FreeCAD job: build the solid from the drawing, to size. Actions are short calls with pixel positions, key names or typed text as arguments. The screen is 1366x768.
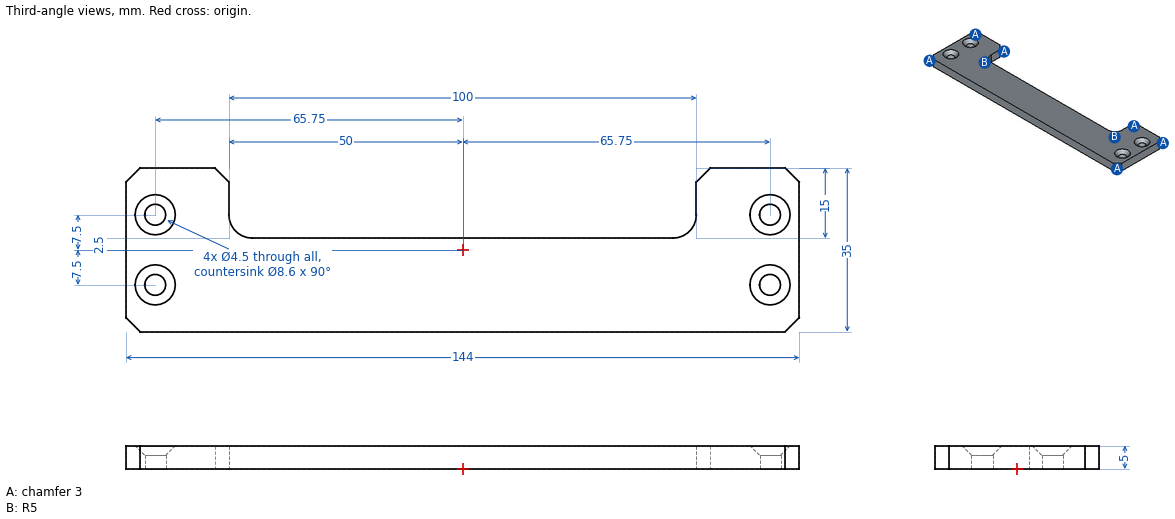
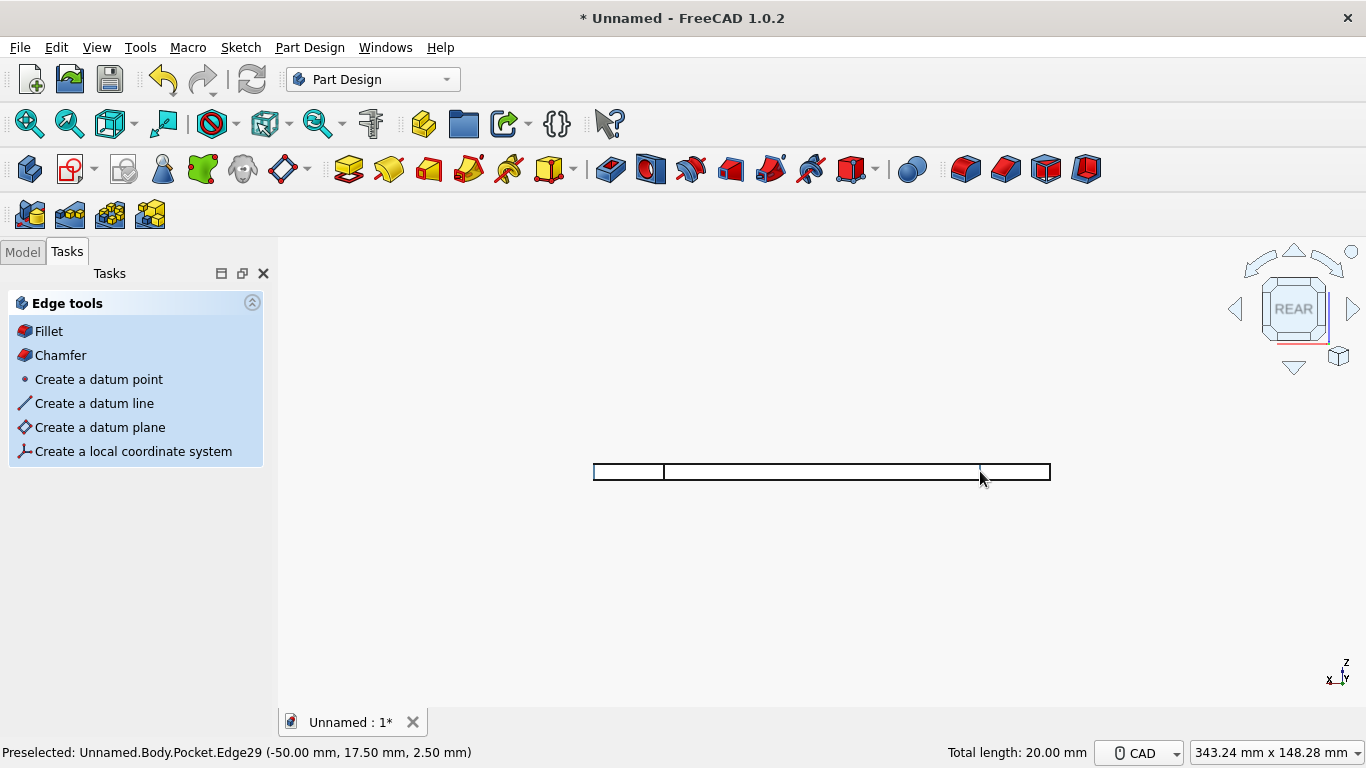
click(664, 471, ctrl)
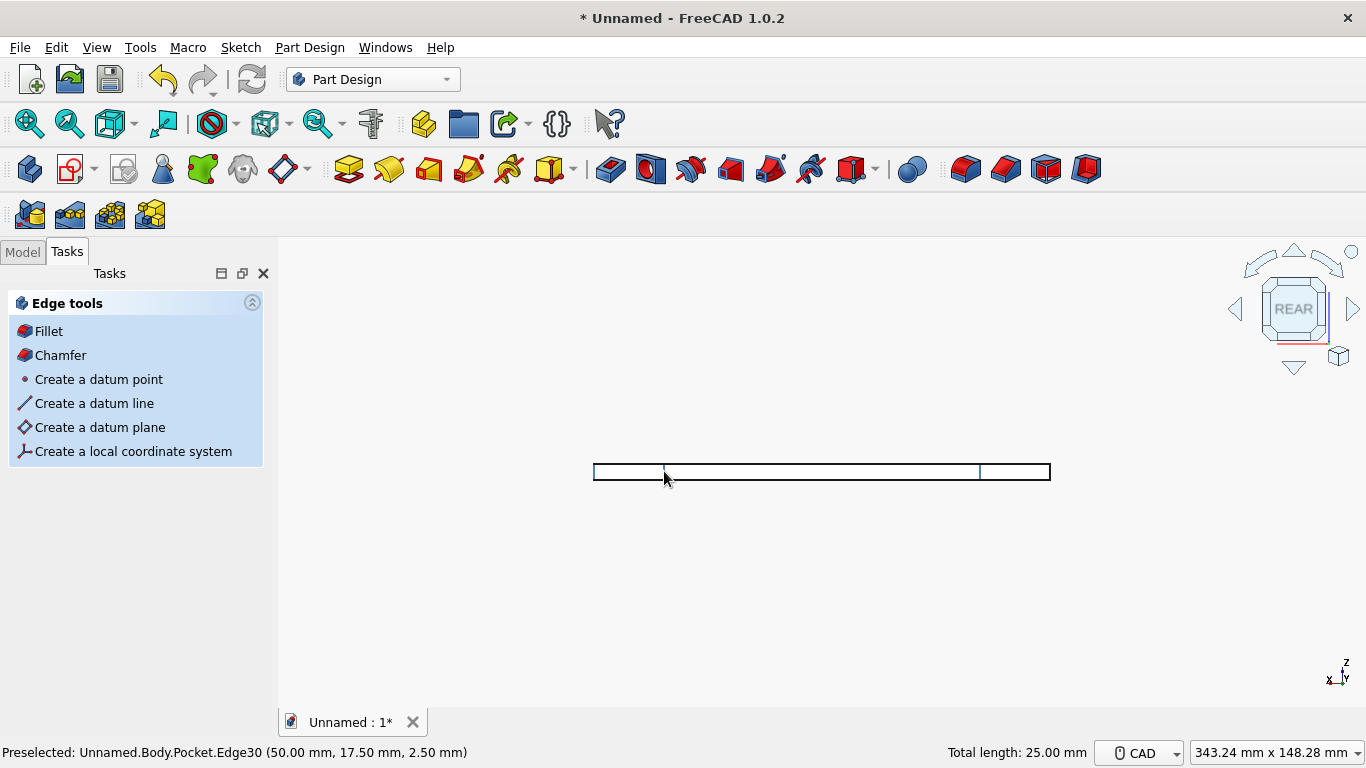
click(1050, 471, ctrl)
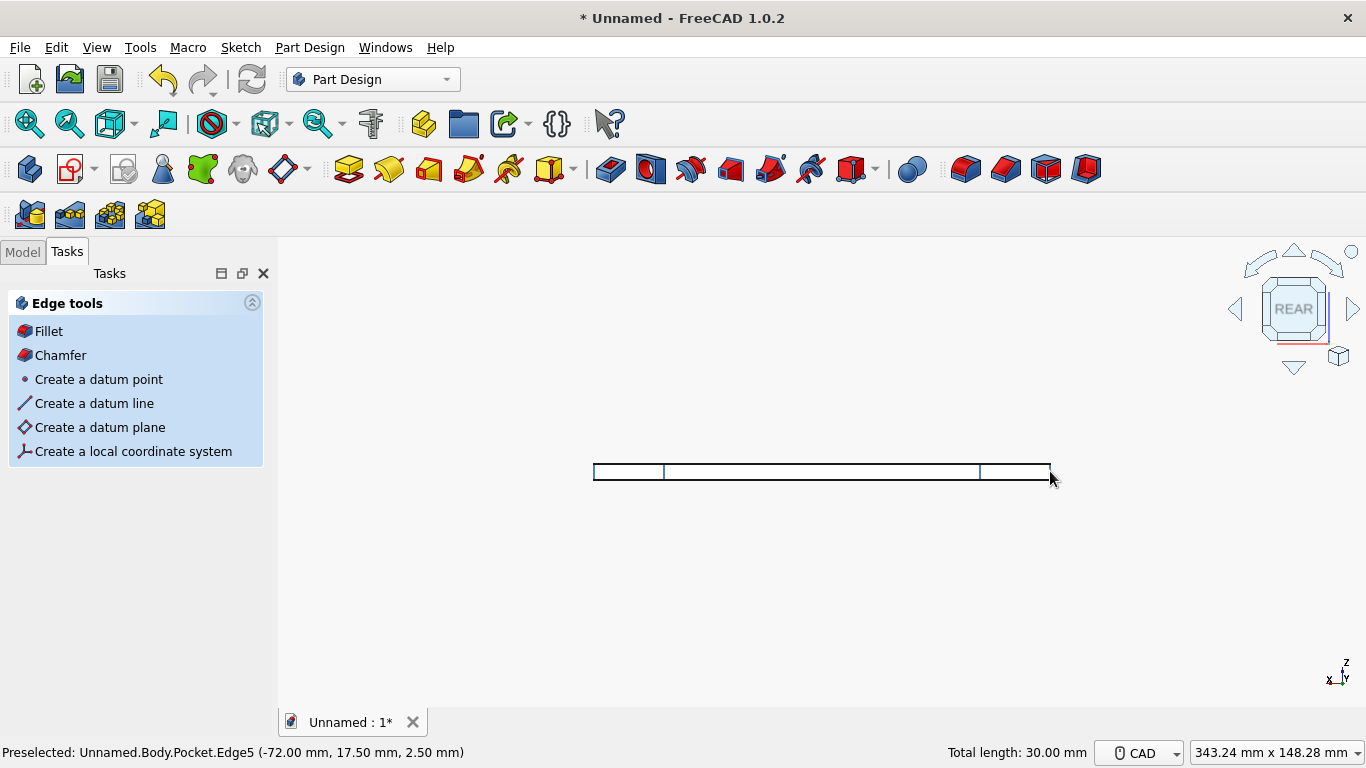
click(1006, 170)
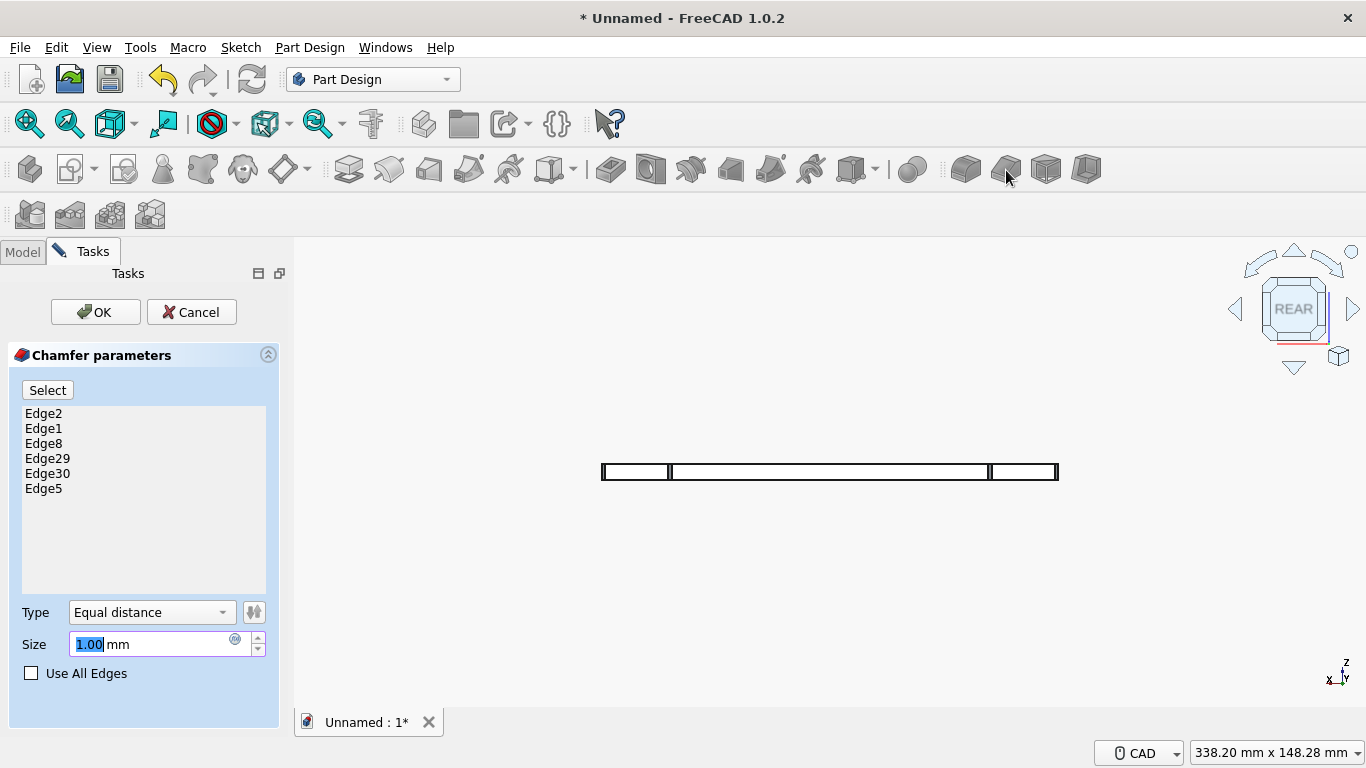
text(3)
key(Tab)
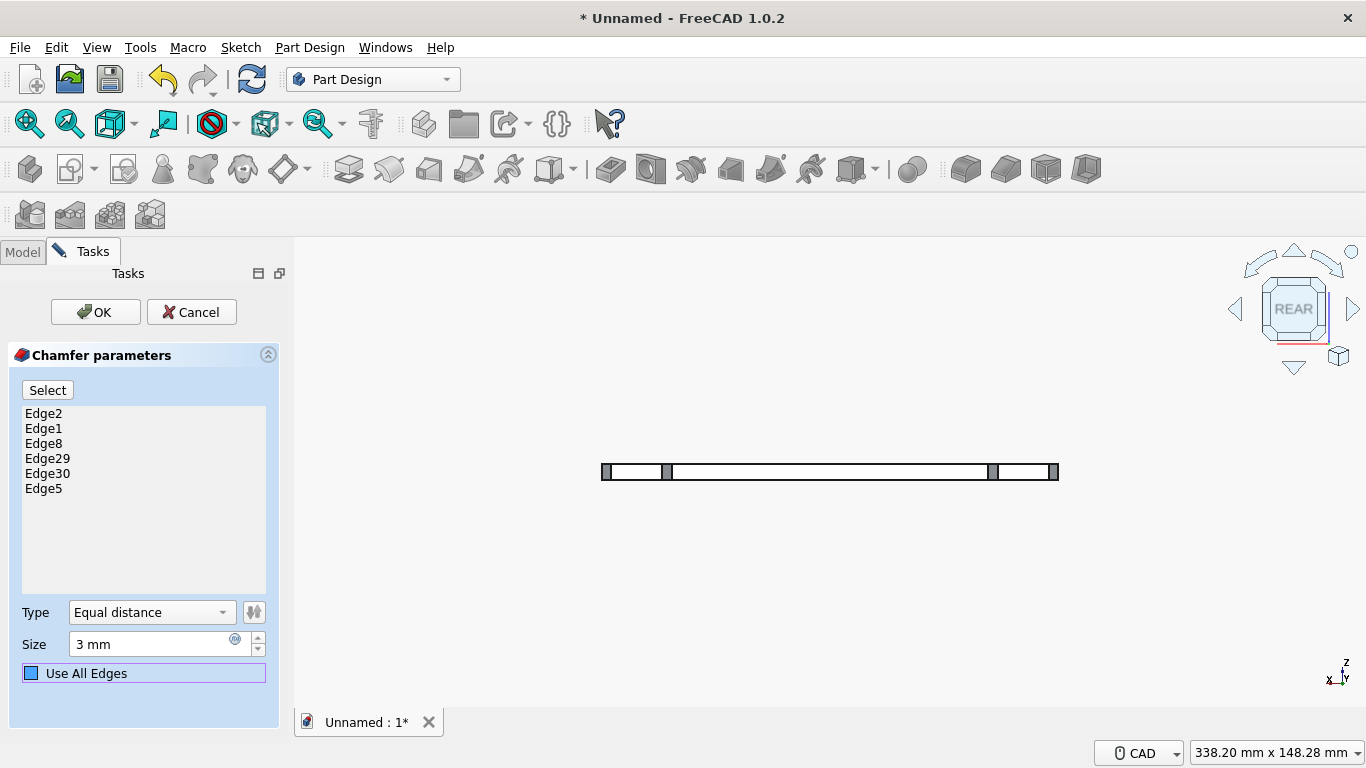
click(96, 312)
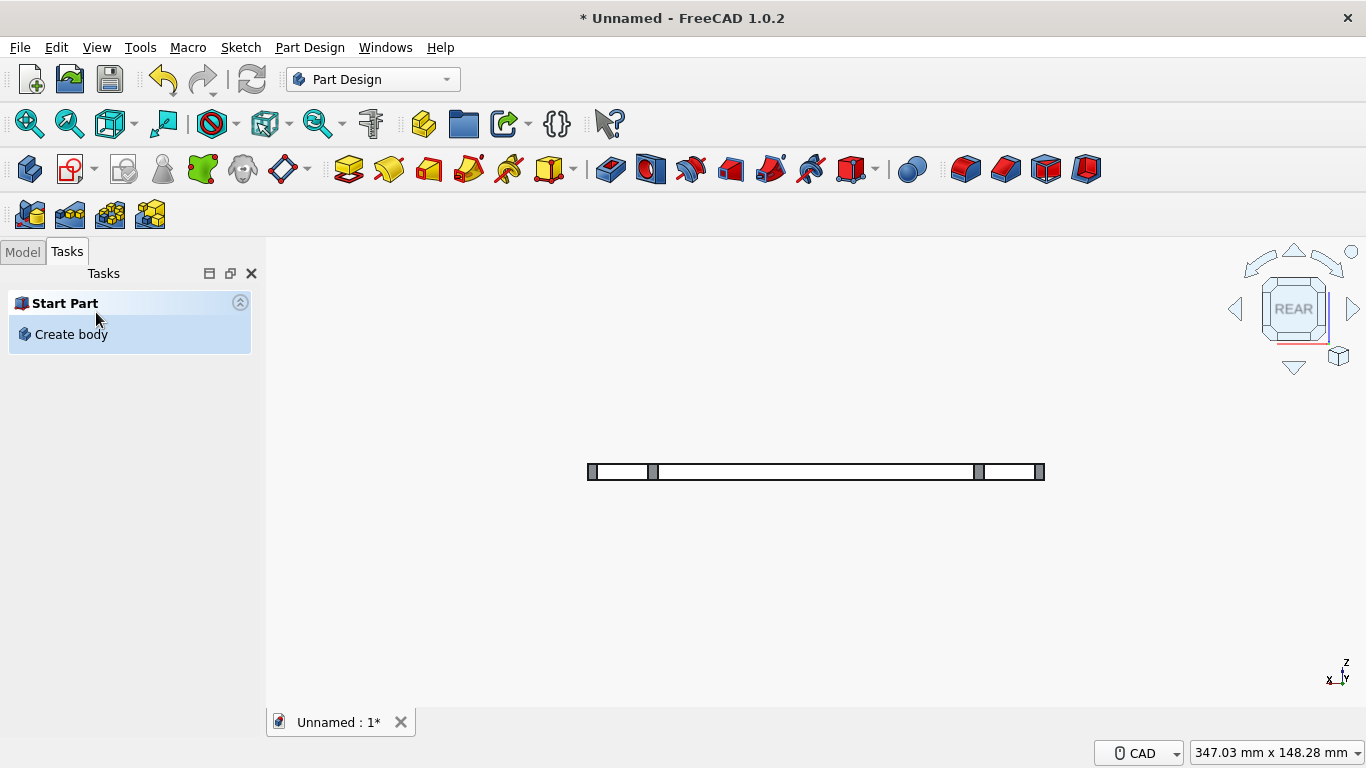
key(v)
key(f)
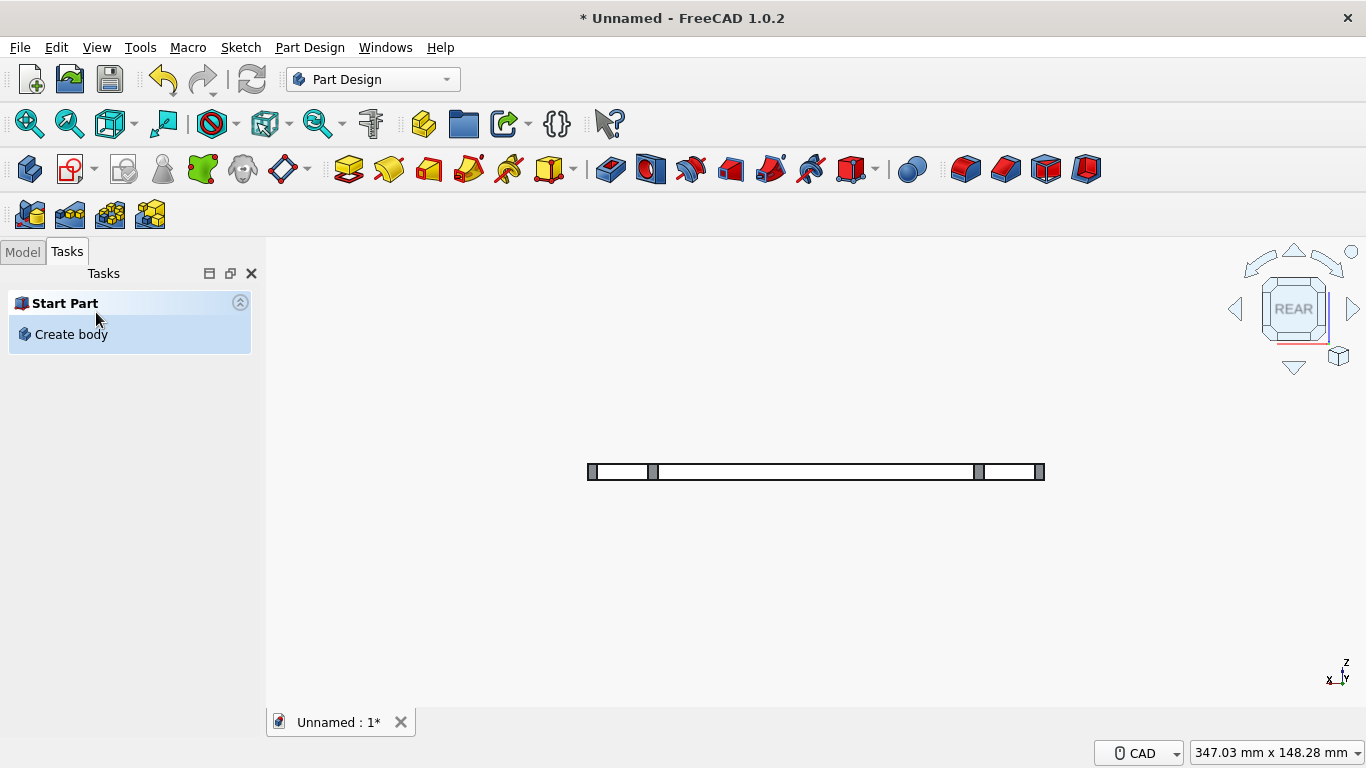
scroll(974, 471, up, 5)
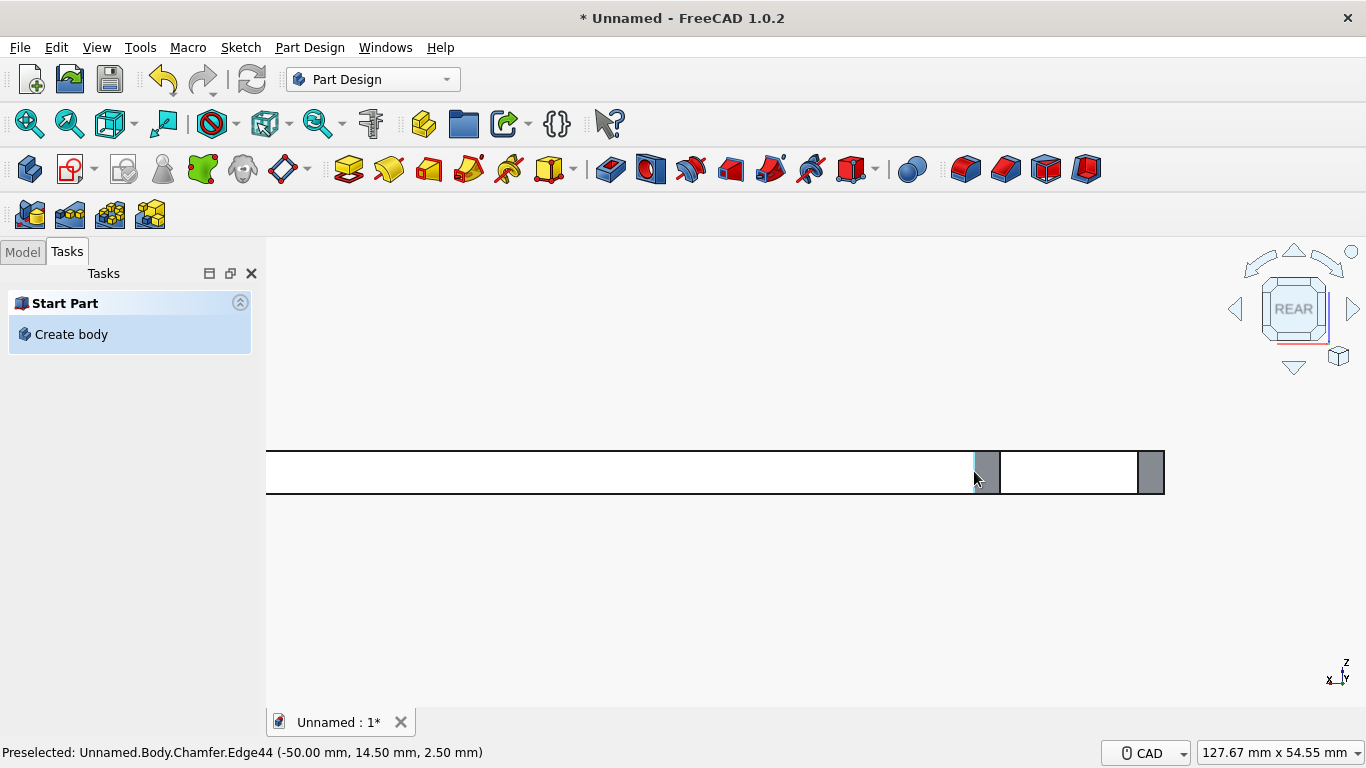
key(v)
key(f)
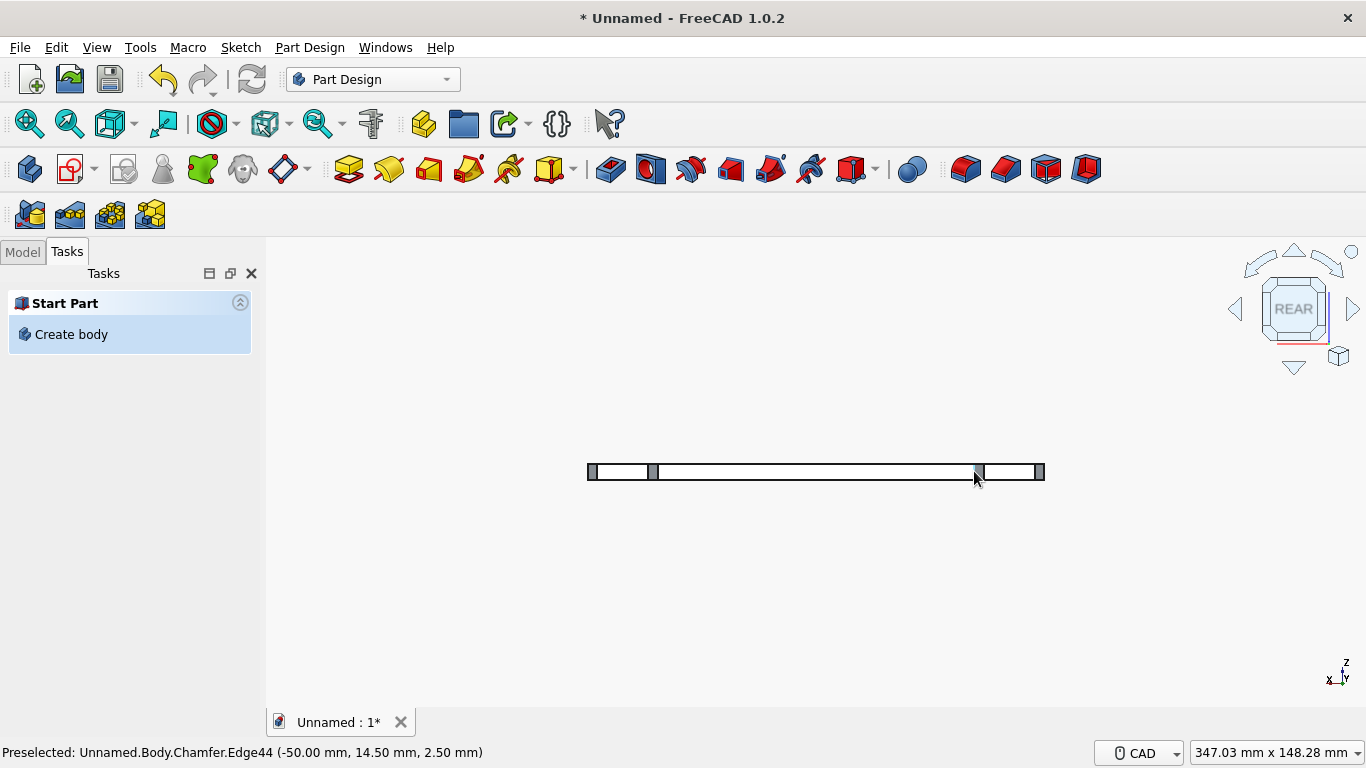
key(0)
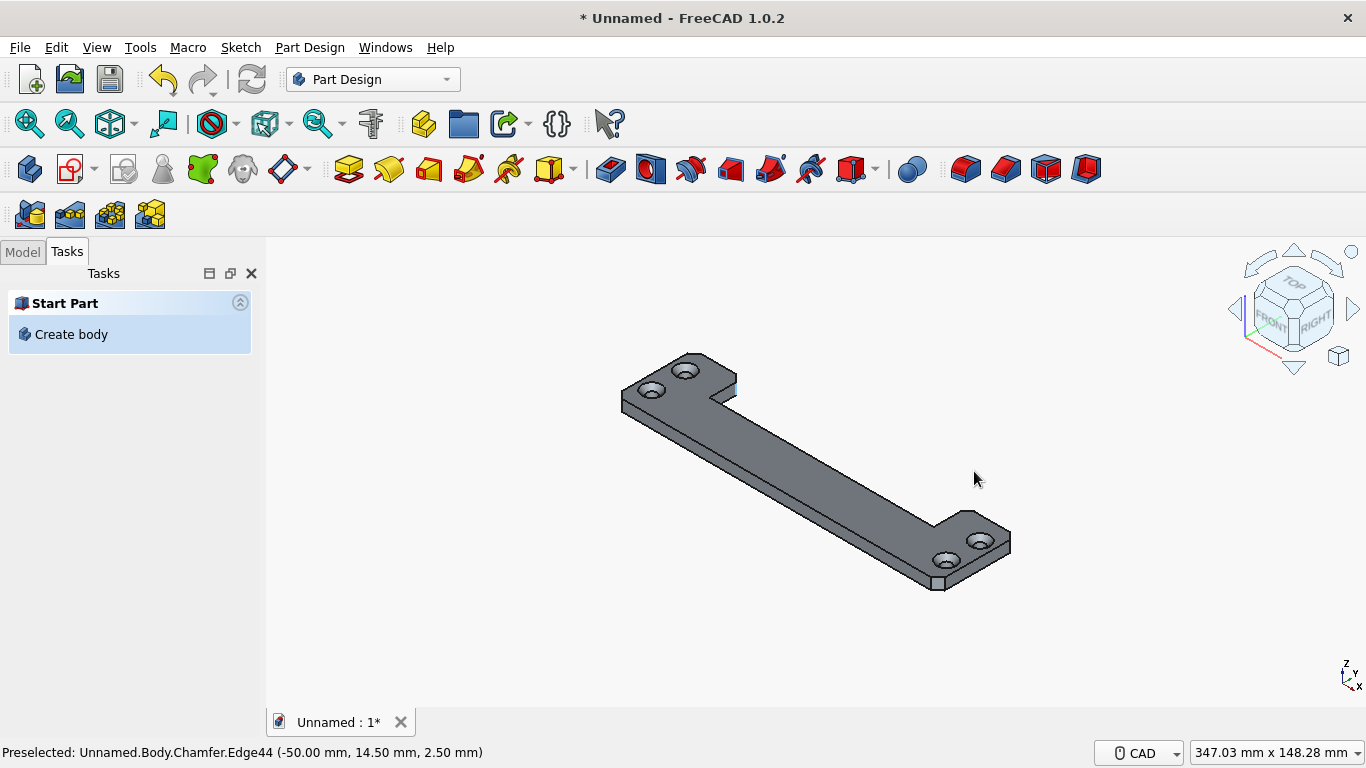
scroll(710, 403, up, 5)